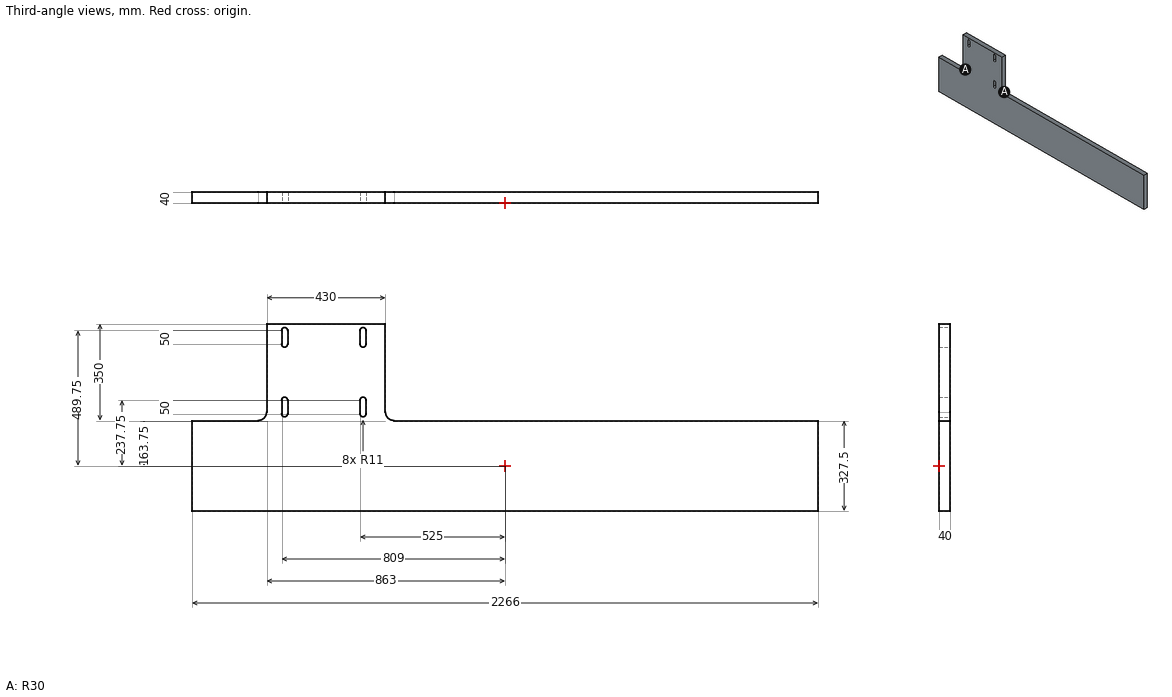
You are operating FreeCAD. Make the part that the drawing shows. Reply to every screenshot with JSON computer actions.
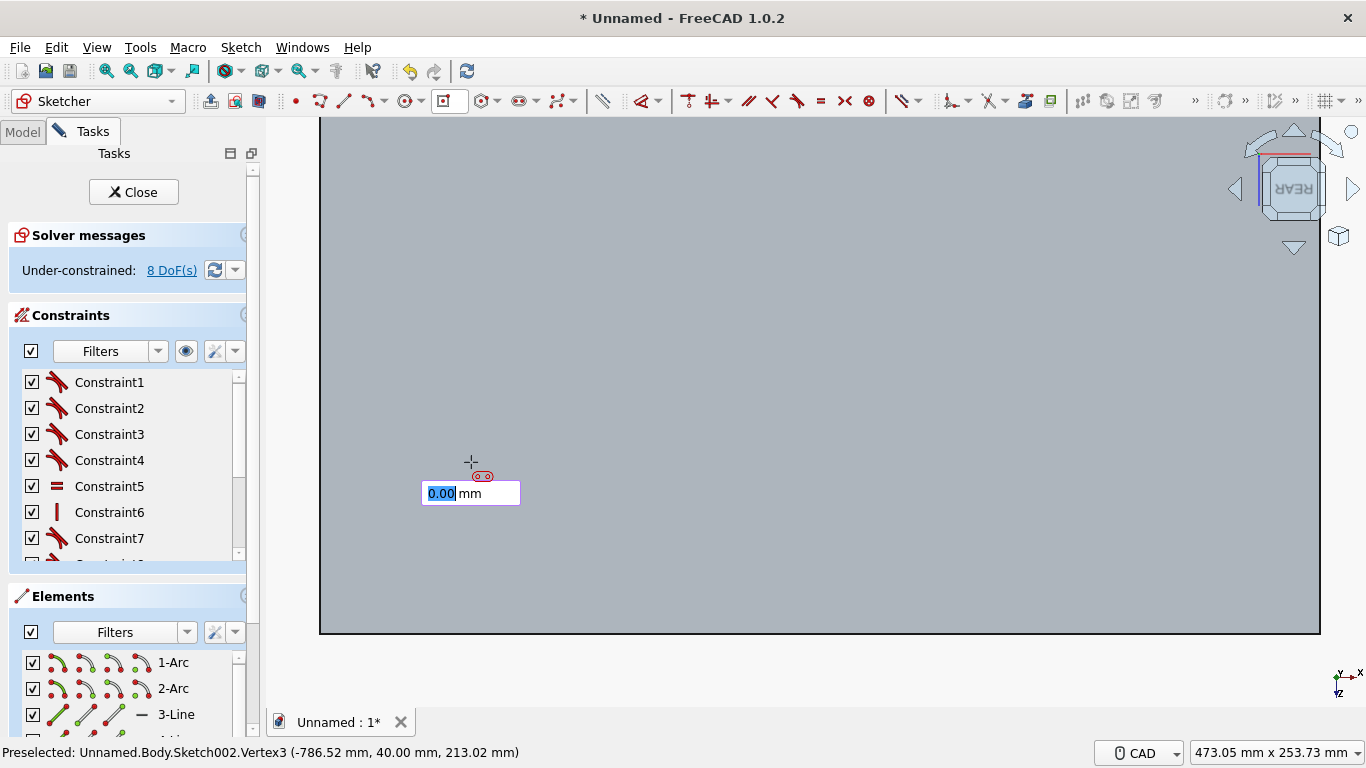
{"action": "left_click", "coordinate": [497, 520]}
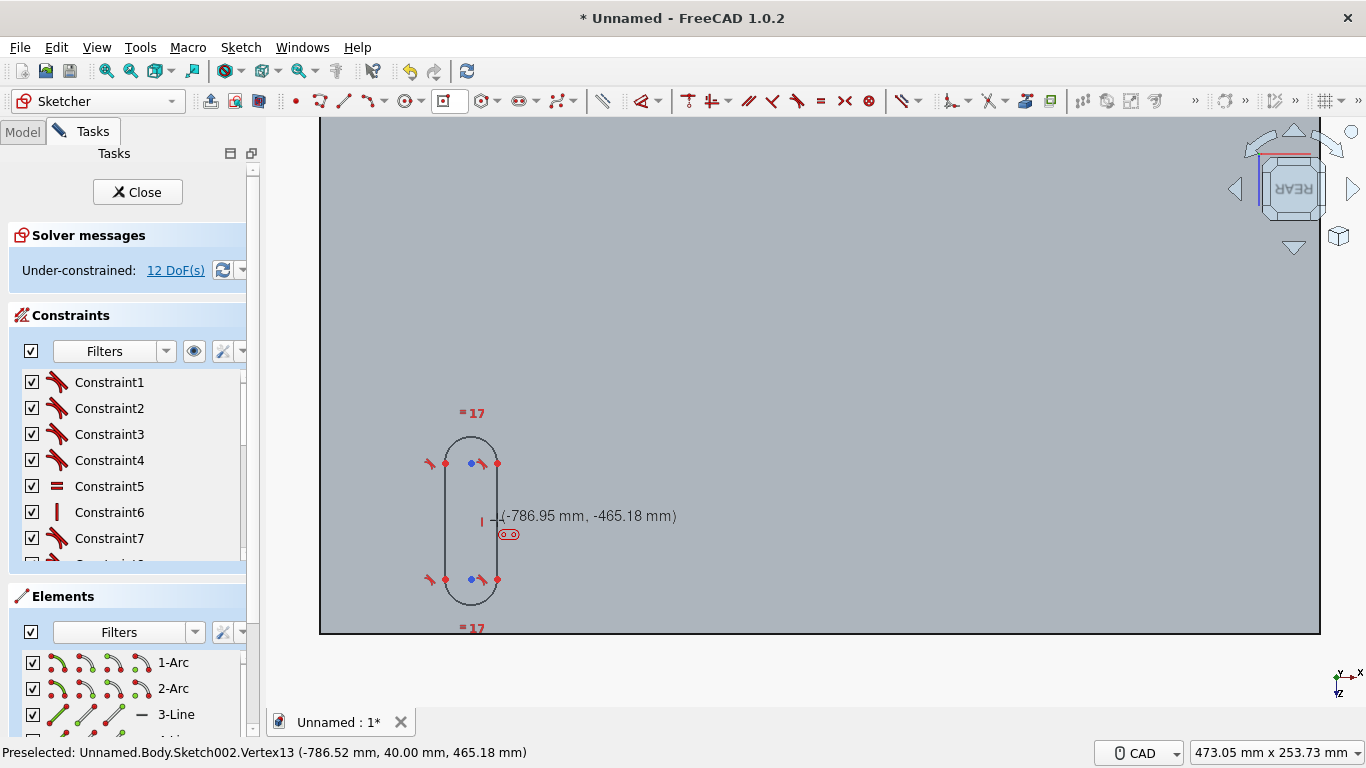
{"action": "left_click", "coordinate": [1132, 578]}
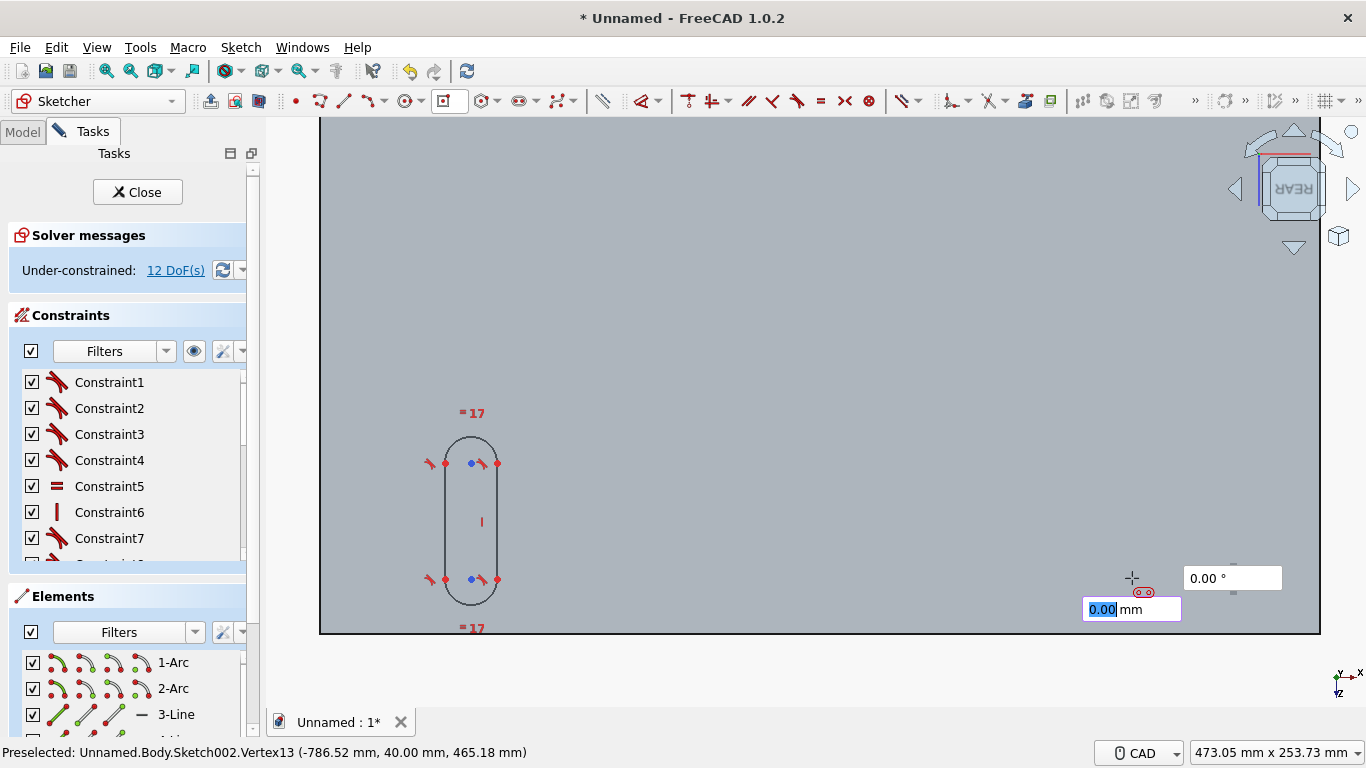
{"action": "left_click", "coordinate": [1132, 462]}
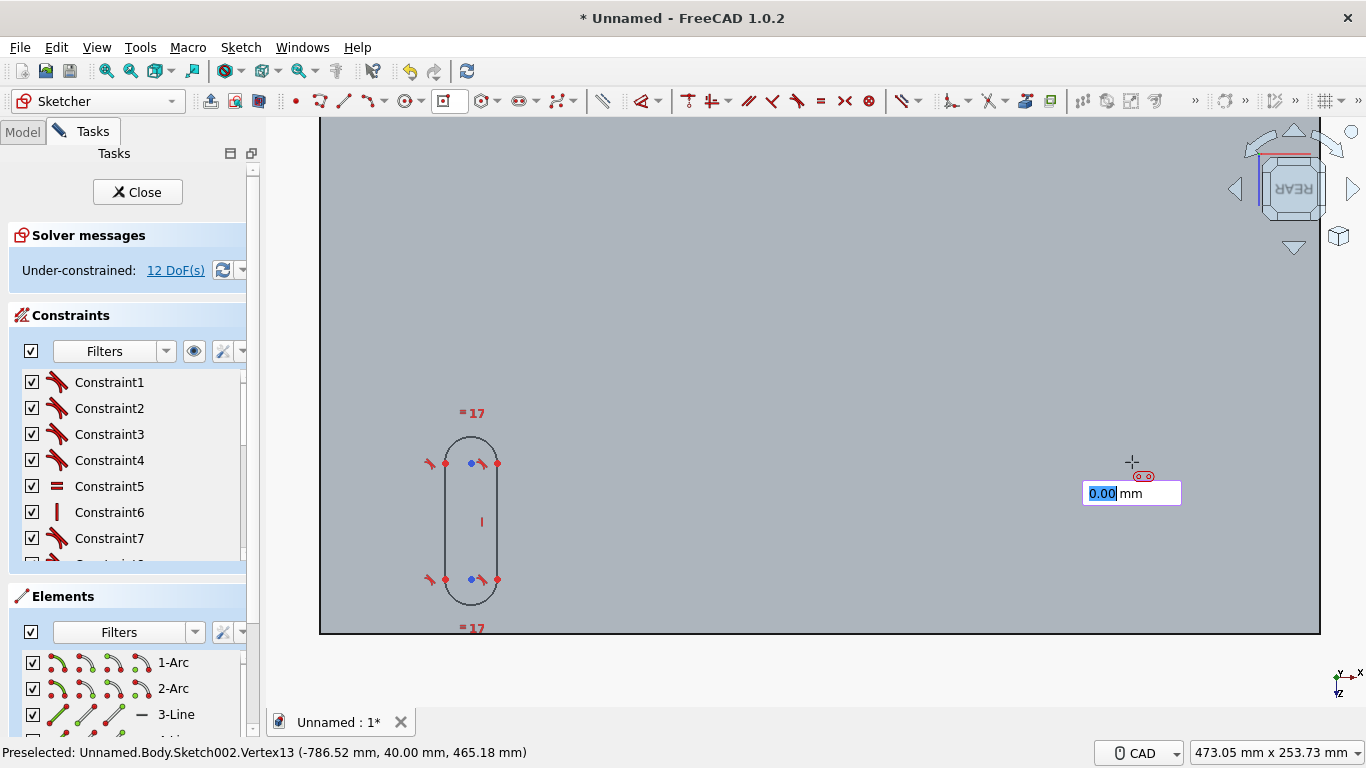
{"action": "left_click", "coordinate": [1157, 520]}
{"action": "key", "text": "Escape"}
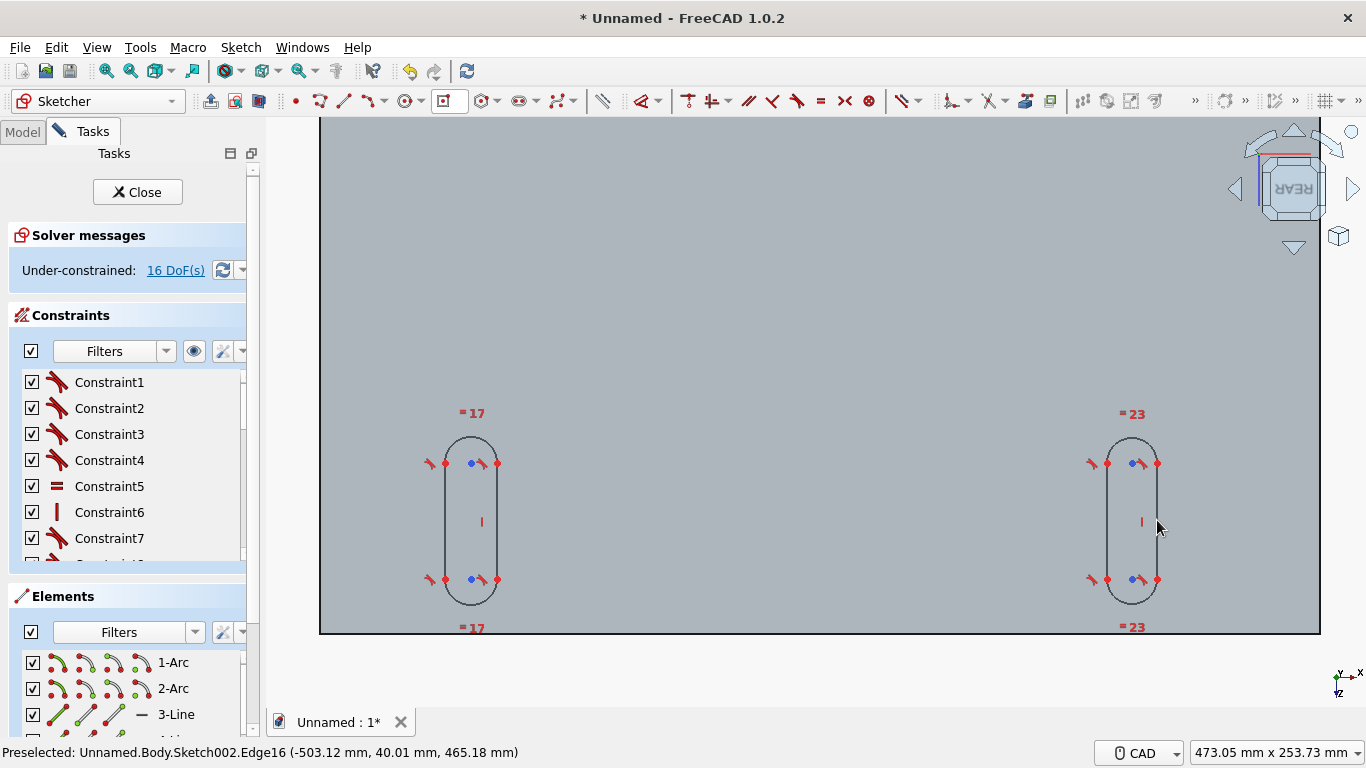
{"action": "scroll", "coordinate": [472, 580], "scroll_direction": "down", "scroll_amount": 6}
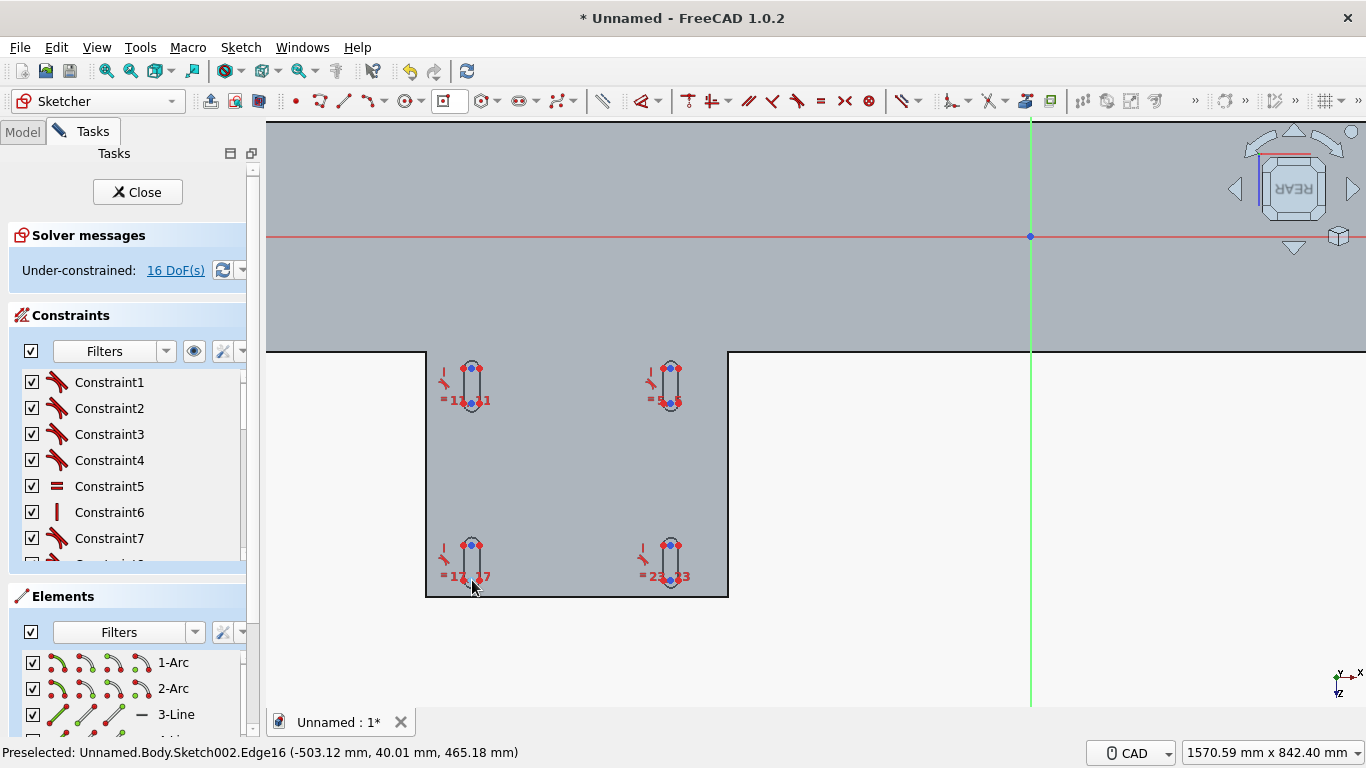
{"action": "scroll", "coordinate": [667, 410], "scroll_direction": "up", "scroll_amount": 4}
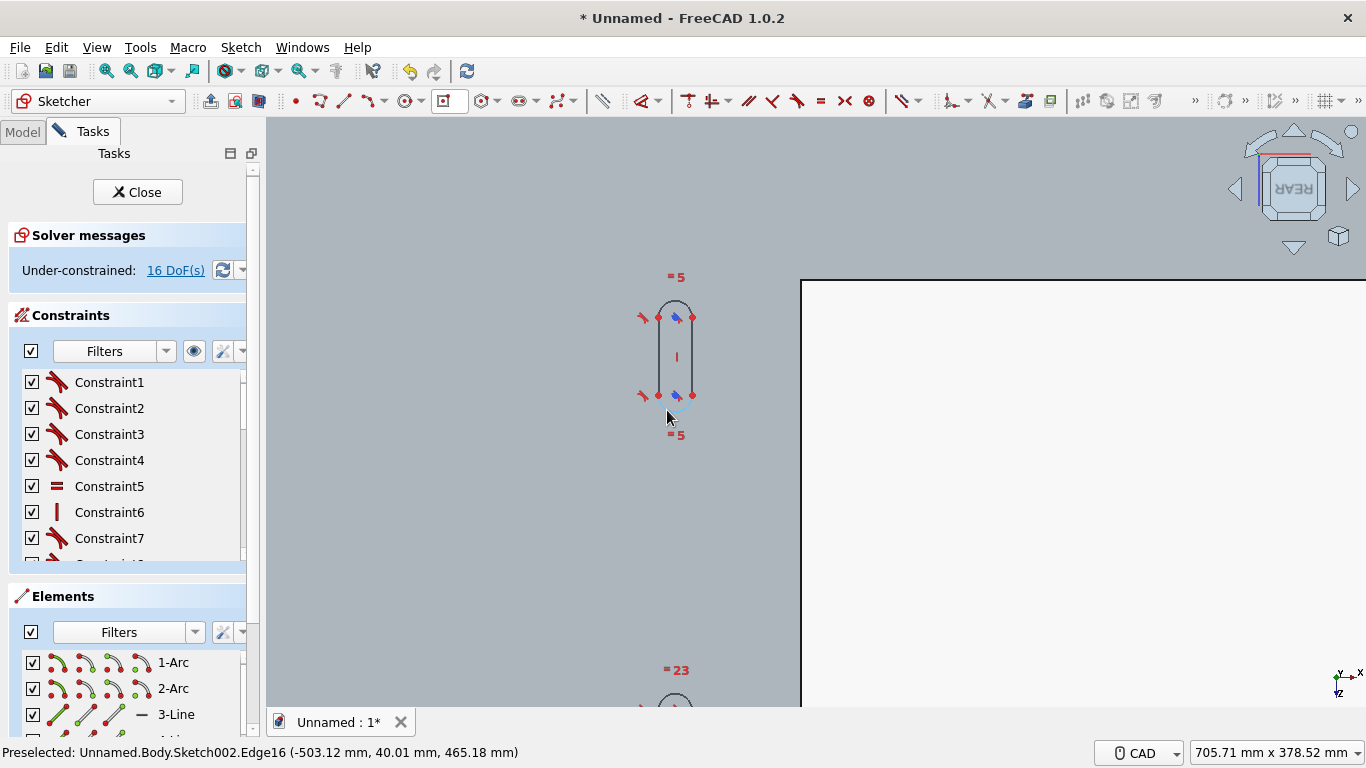
{"action": "left_click", "coordinate": [666, 409]}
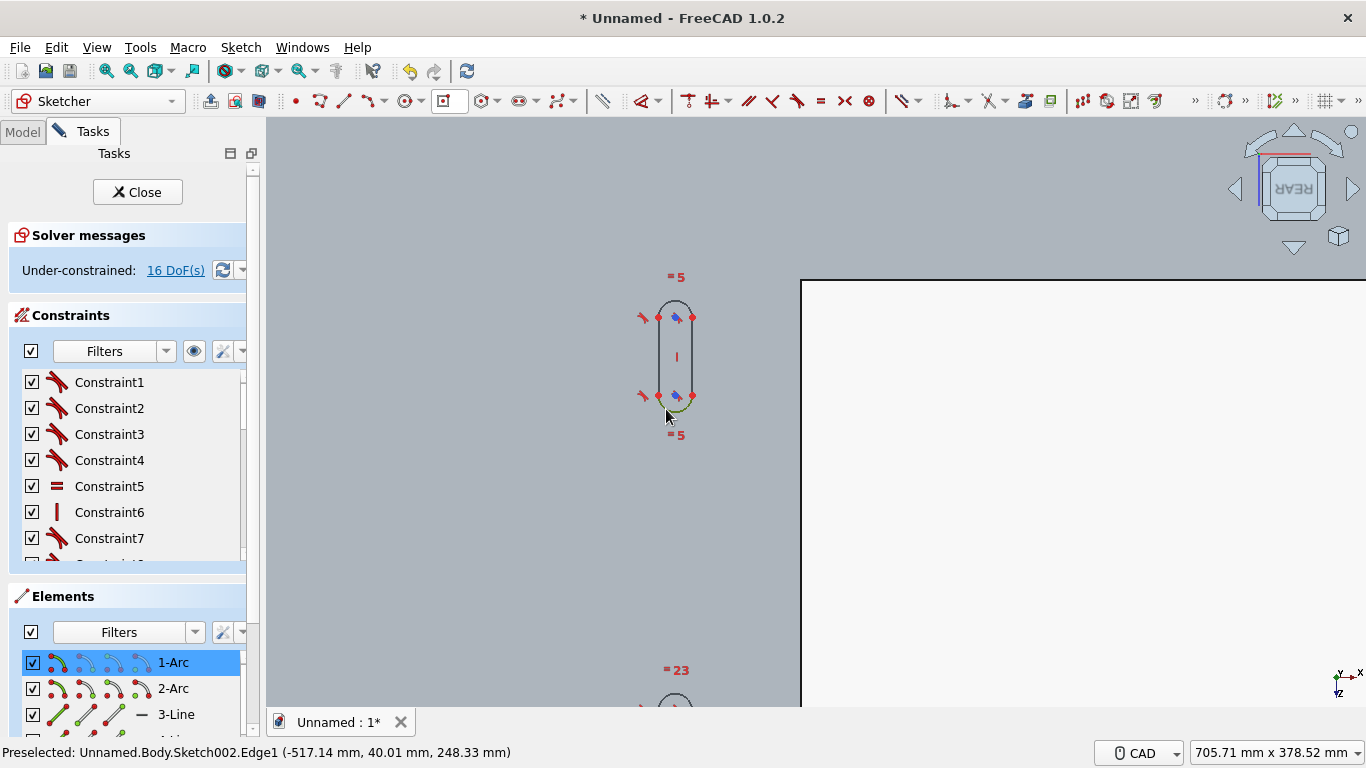
{"action": "scroll", "coordinate": [667, 410], "scroll_direction": "down", "scroll_amount": 4}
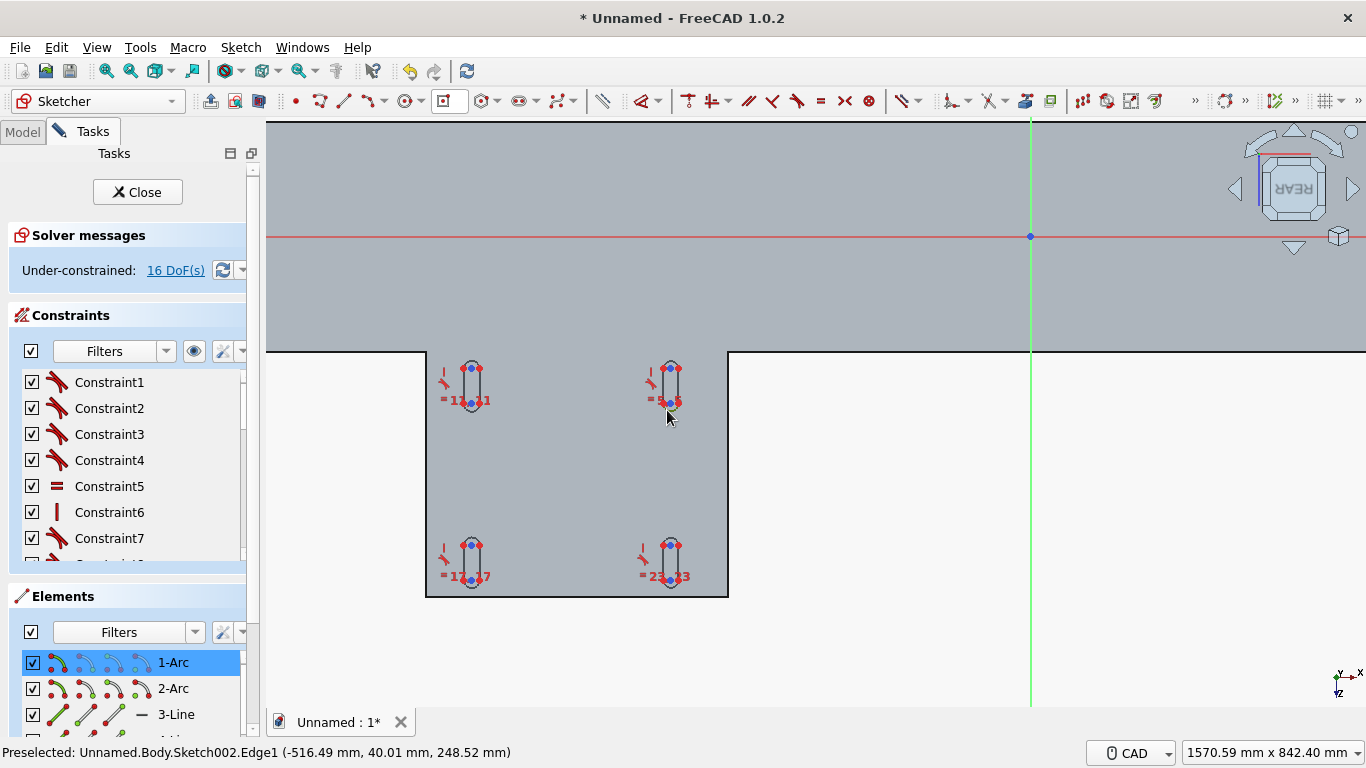
{"action": "scroll", "coordinate": [467, 410], "scroll_direction": "up", "scroll_amount": 4}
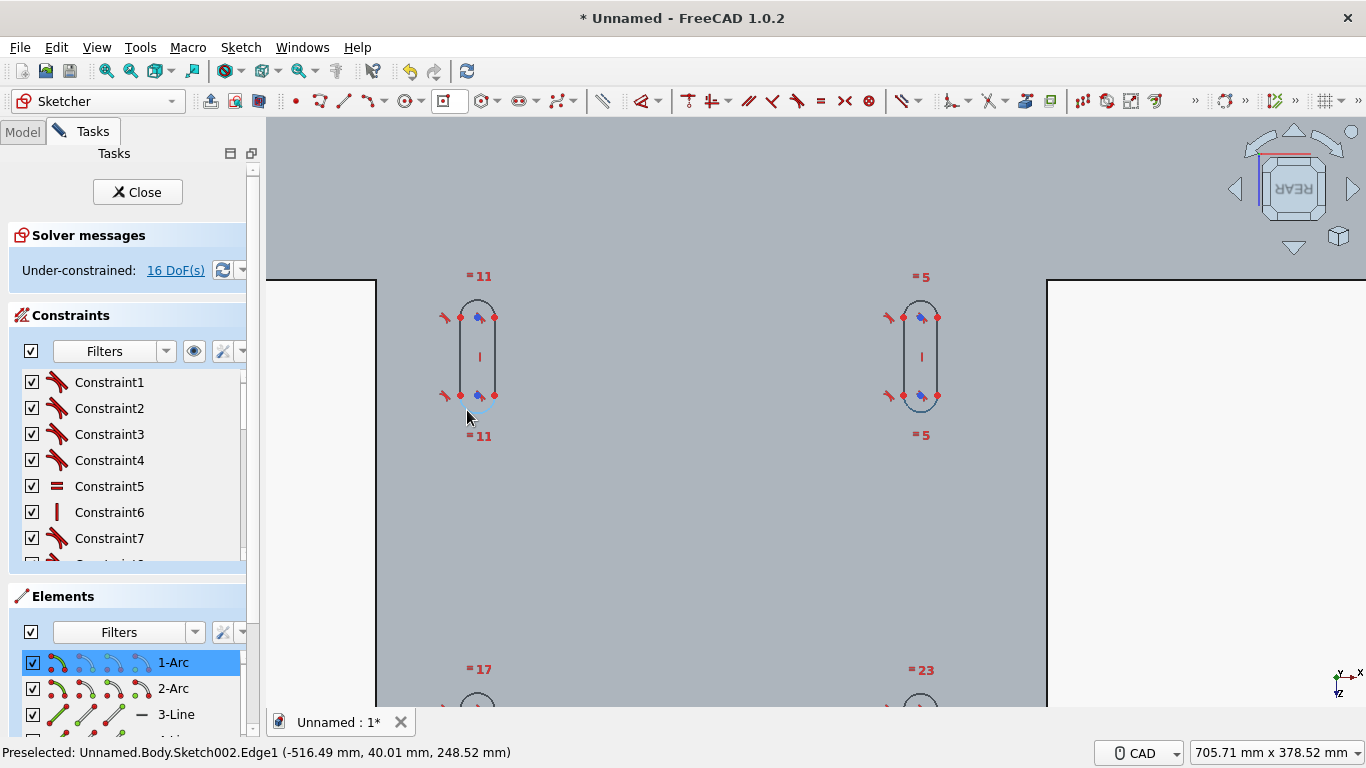
{"action": "left_click", "coordinate": [467, 410]}